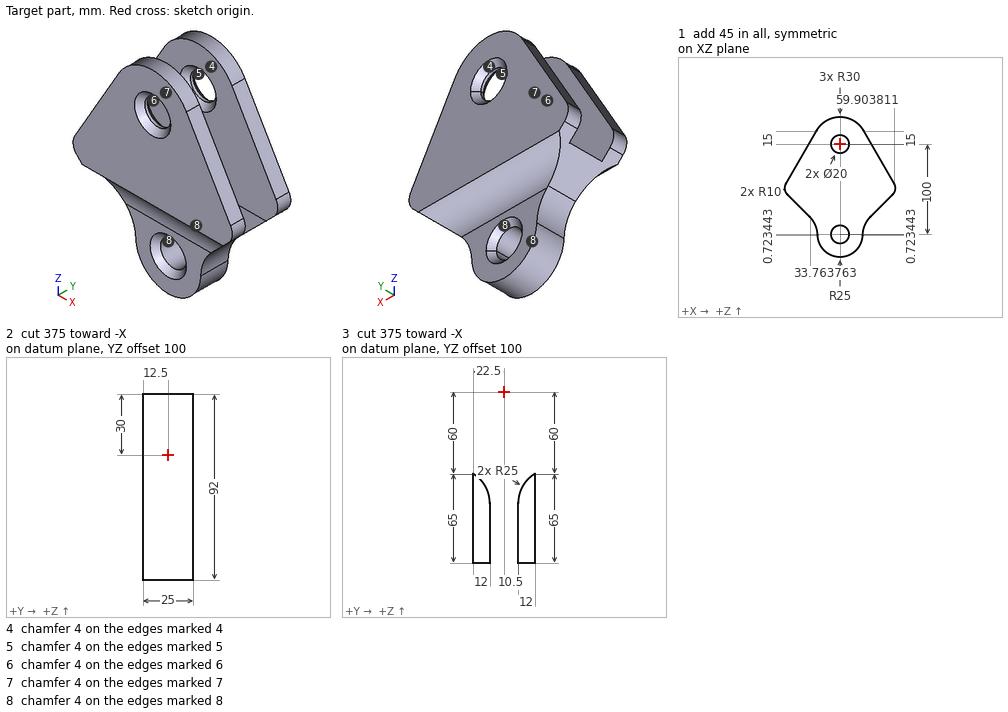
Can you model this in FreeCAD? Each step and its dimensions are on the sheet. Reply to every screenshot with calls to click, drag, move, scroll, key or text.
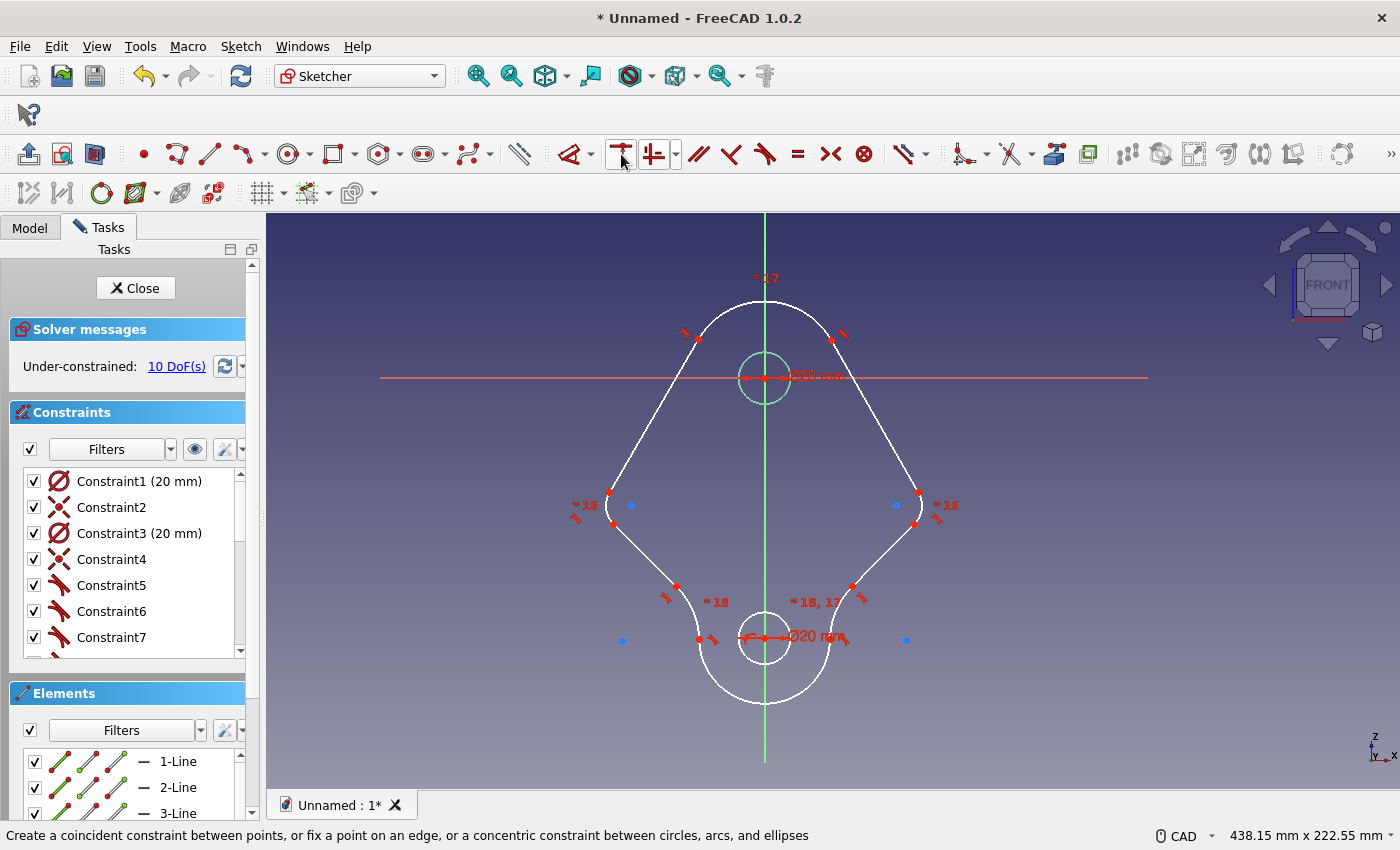
key(d)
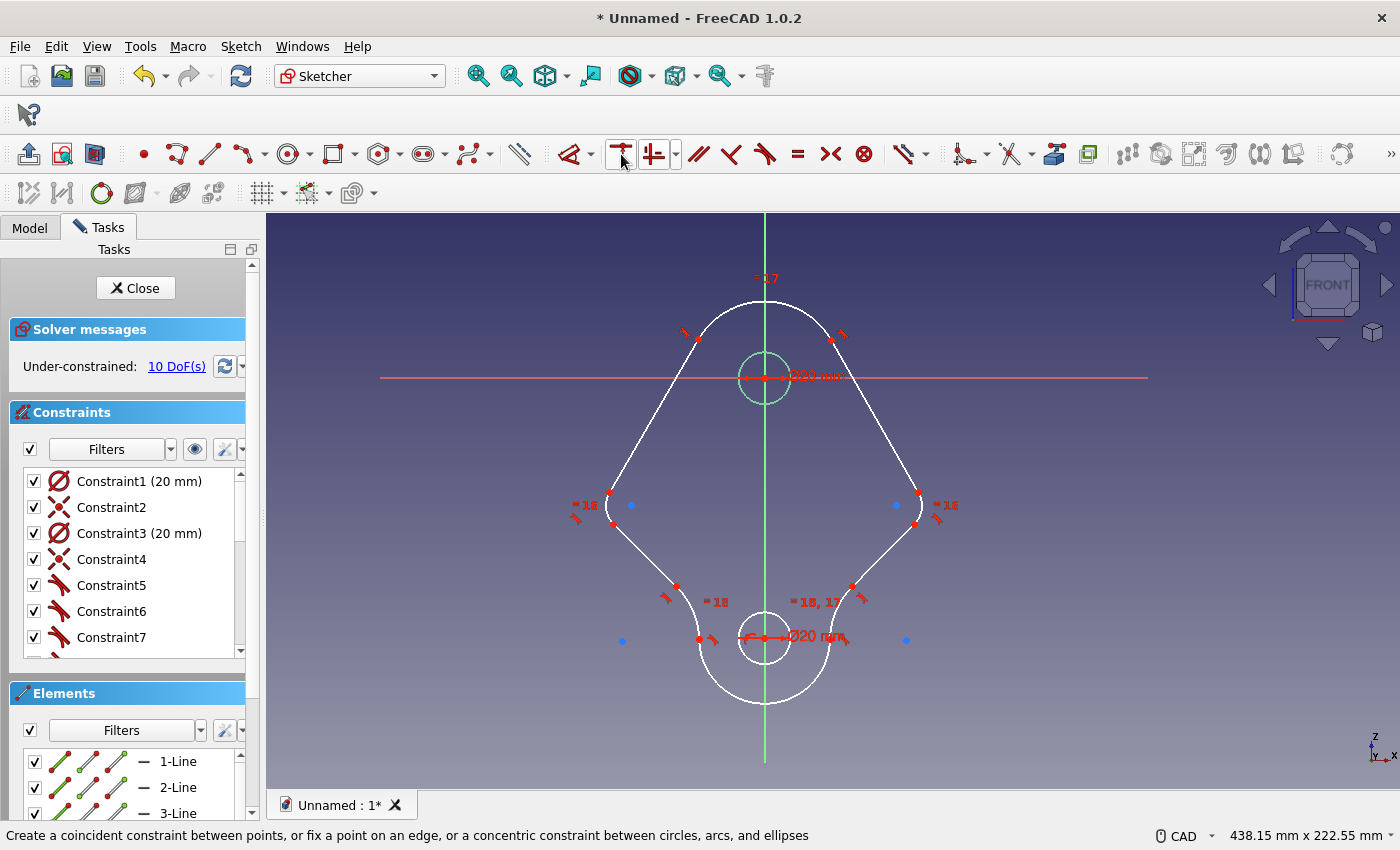
scroll(606, 502, up, 3)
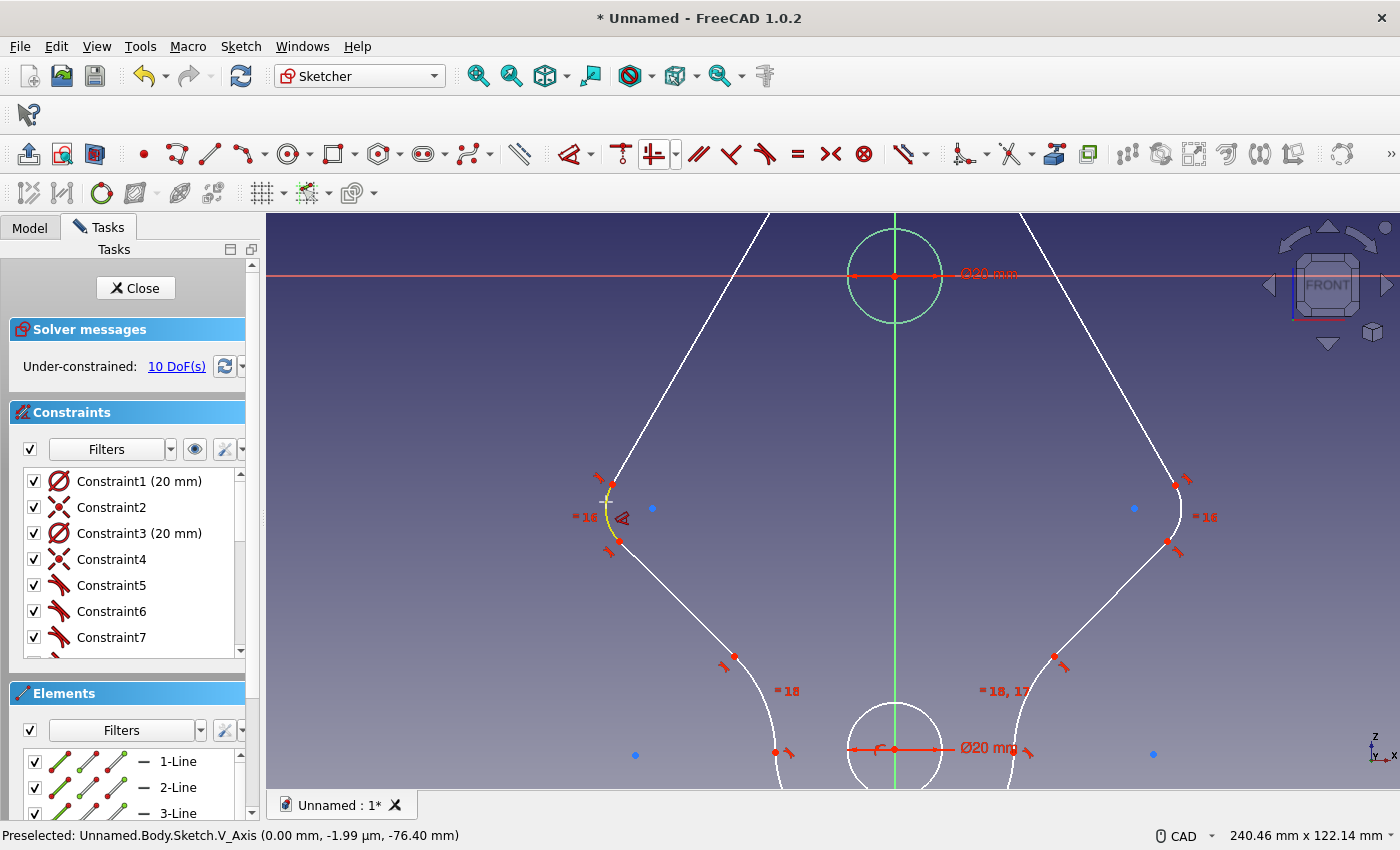
click(606, 502)
click(574, 498)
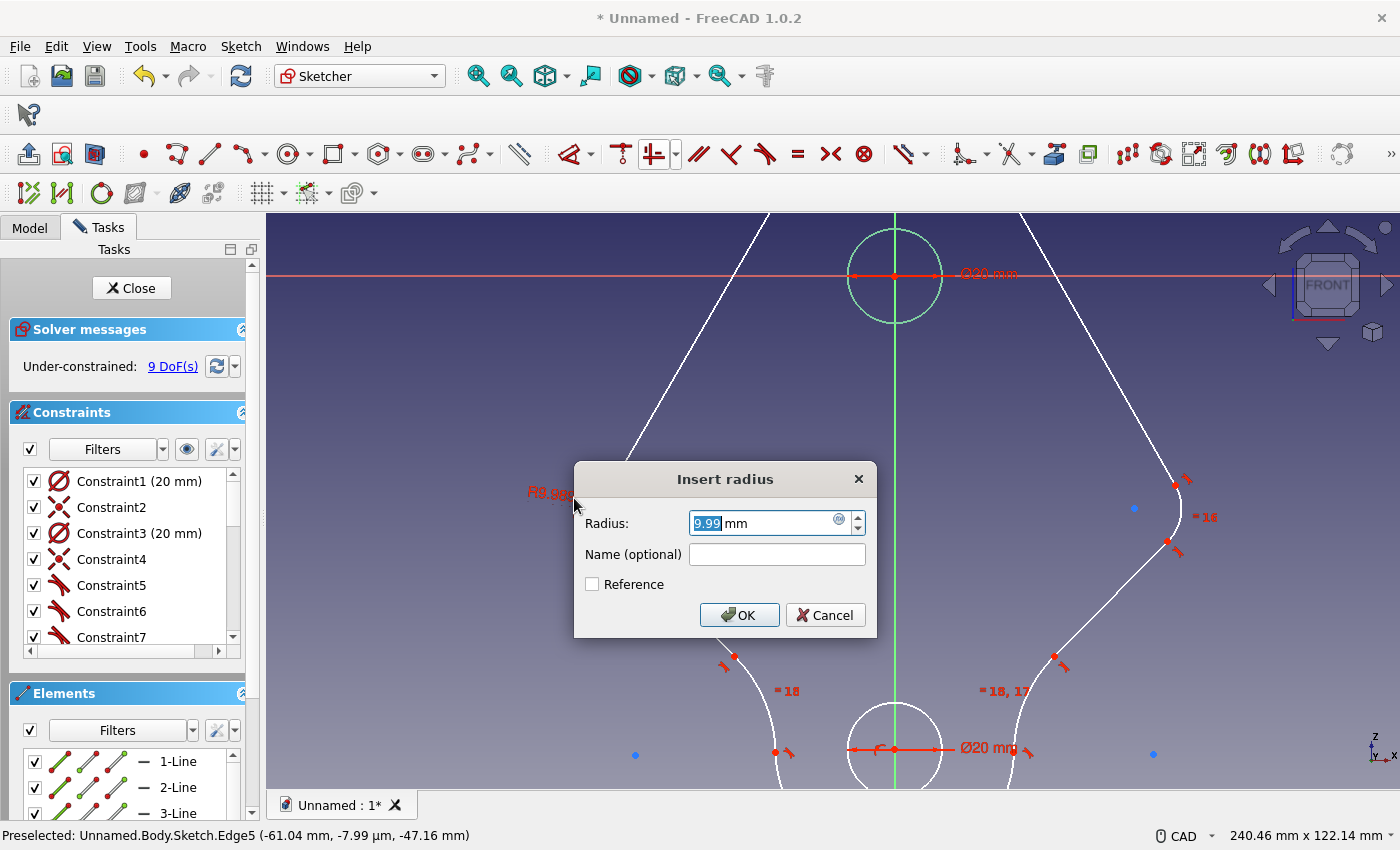
text(10)
key(Return)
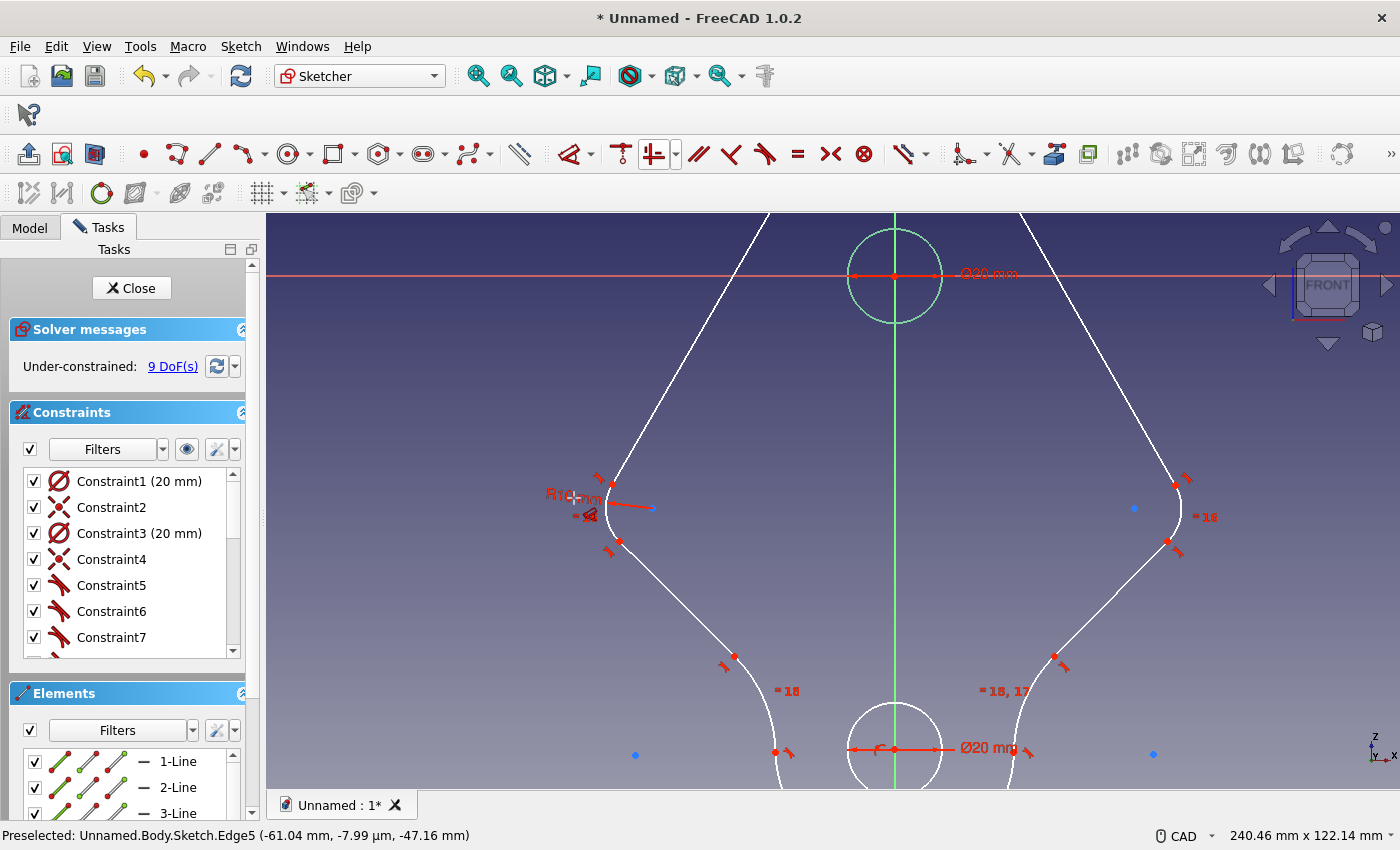
scroll(606, 502, down, 3)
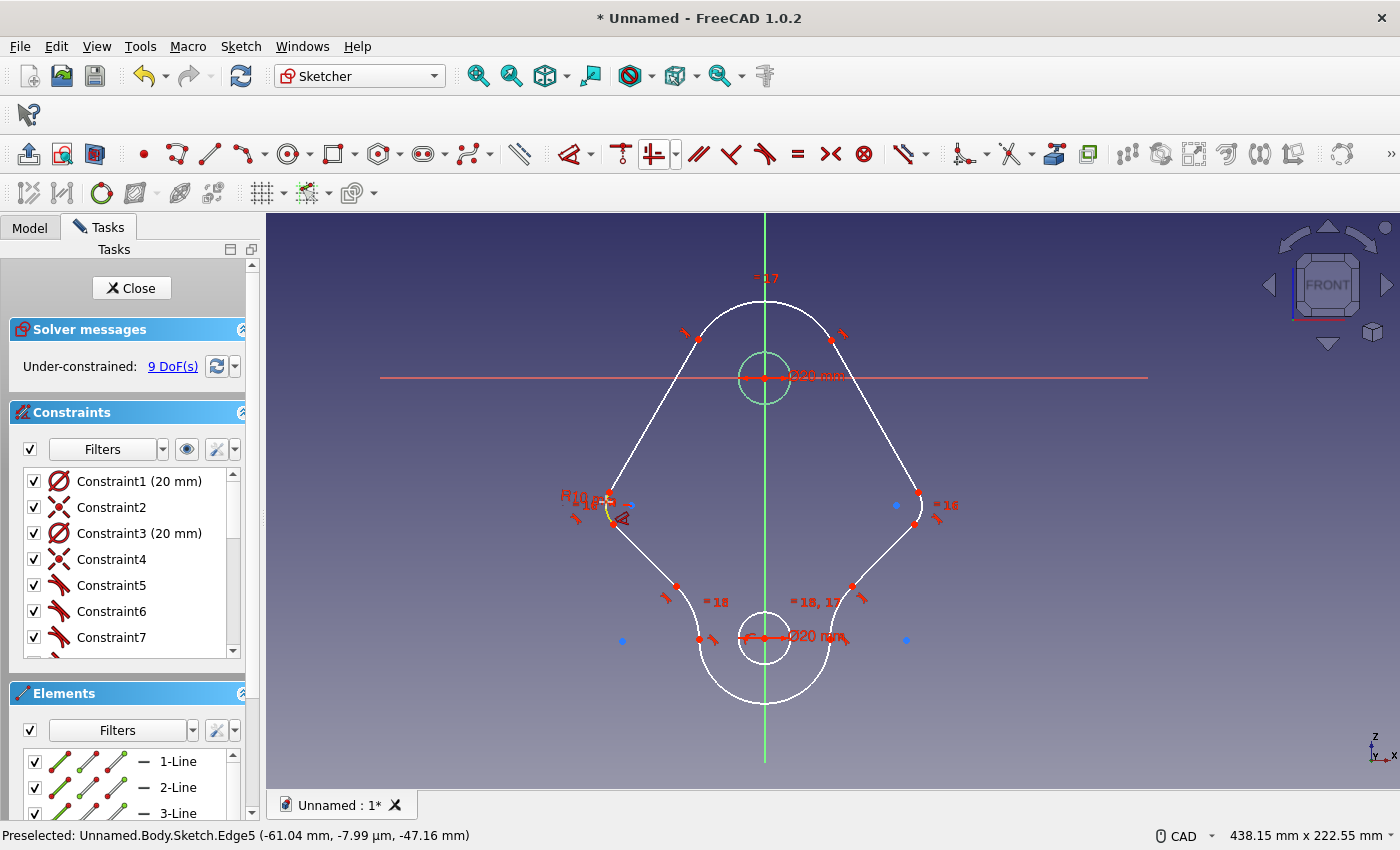
click(796, 308)
click(809, 279)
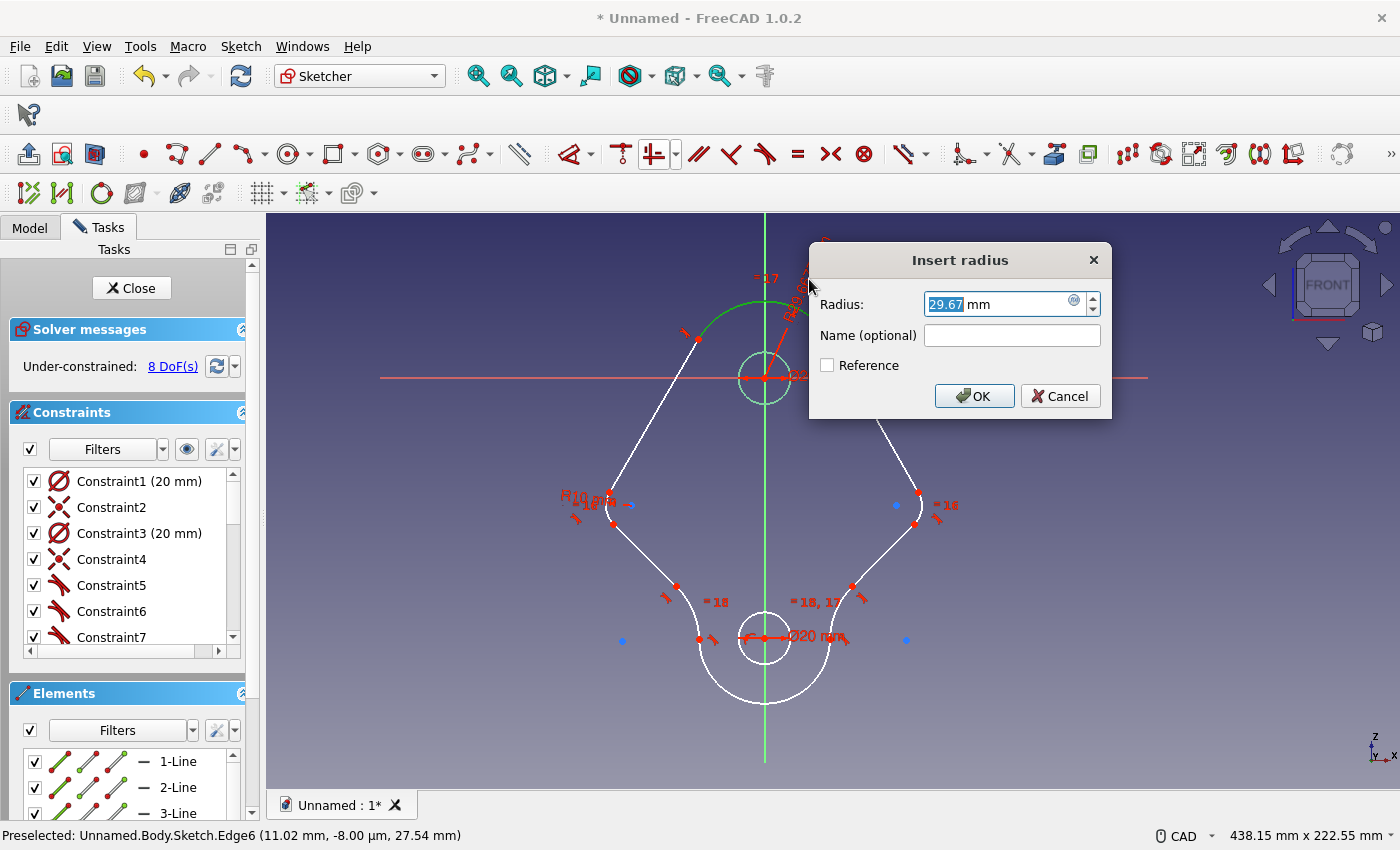
text(30)
key(Return)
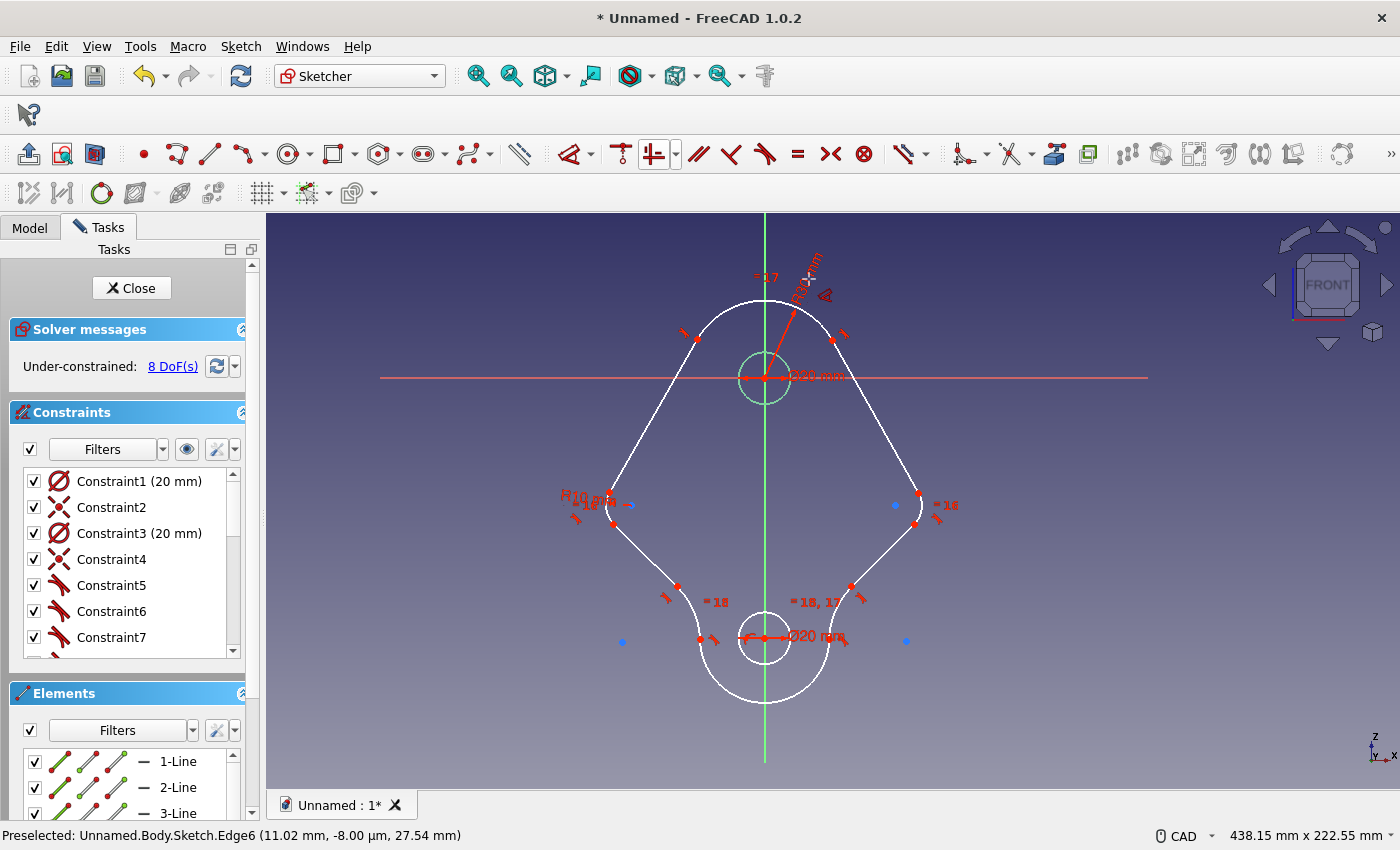
click(727, 691)
click(708, 717)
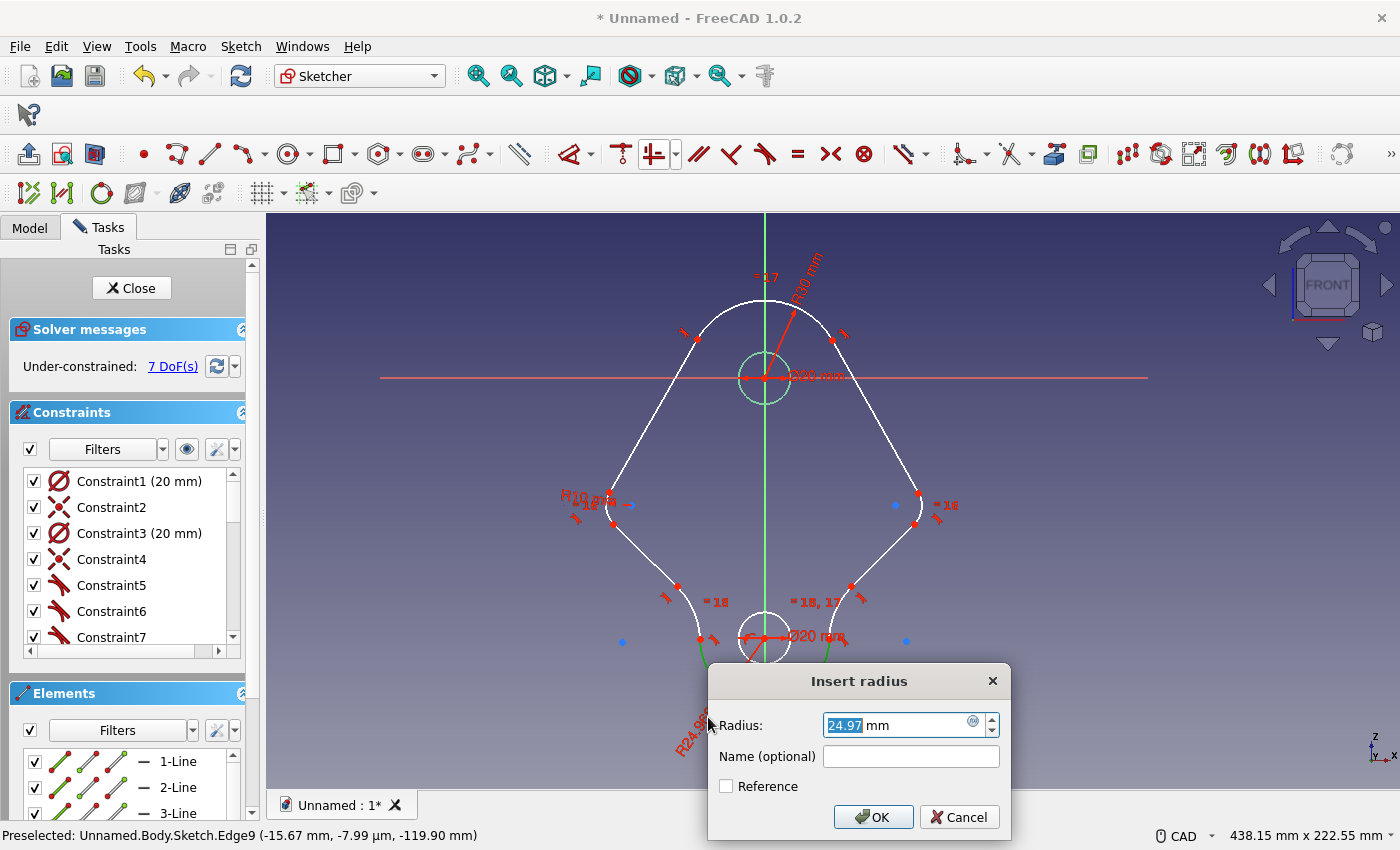
text(25)
key(Return)